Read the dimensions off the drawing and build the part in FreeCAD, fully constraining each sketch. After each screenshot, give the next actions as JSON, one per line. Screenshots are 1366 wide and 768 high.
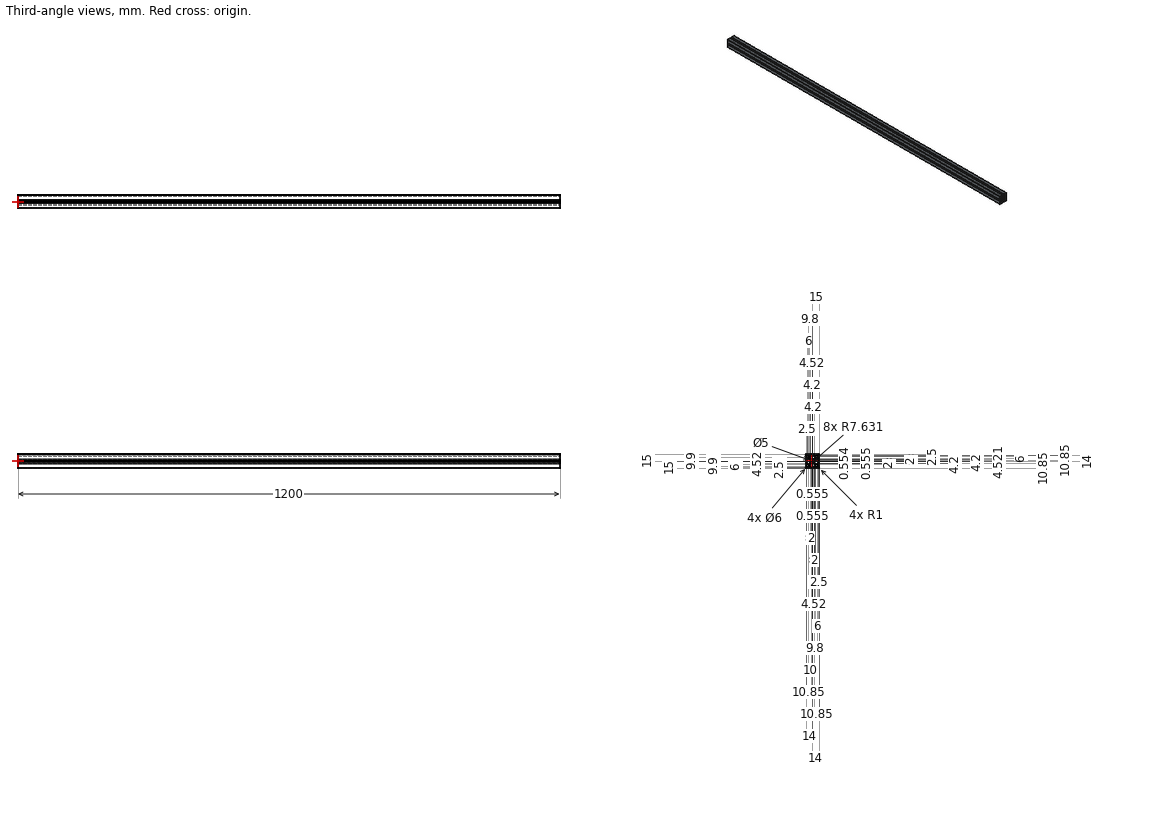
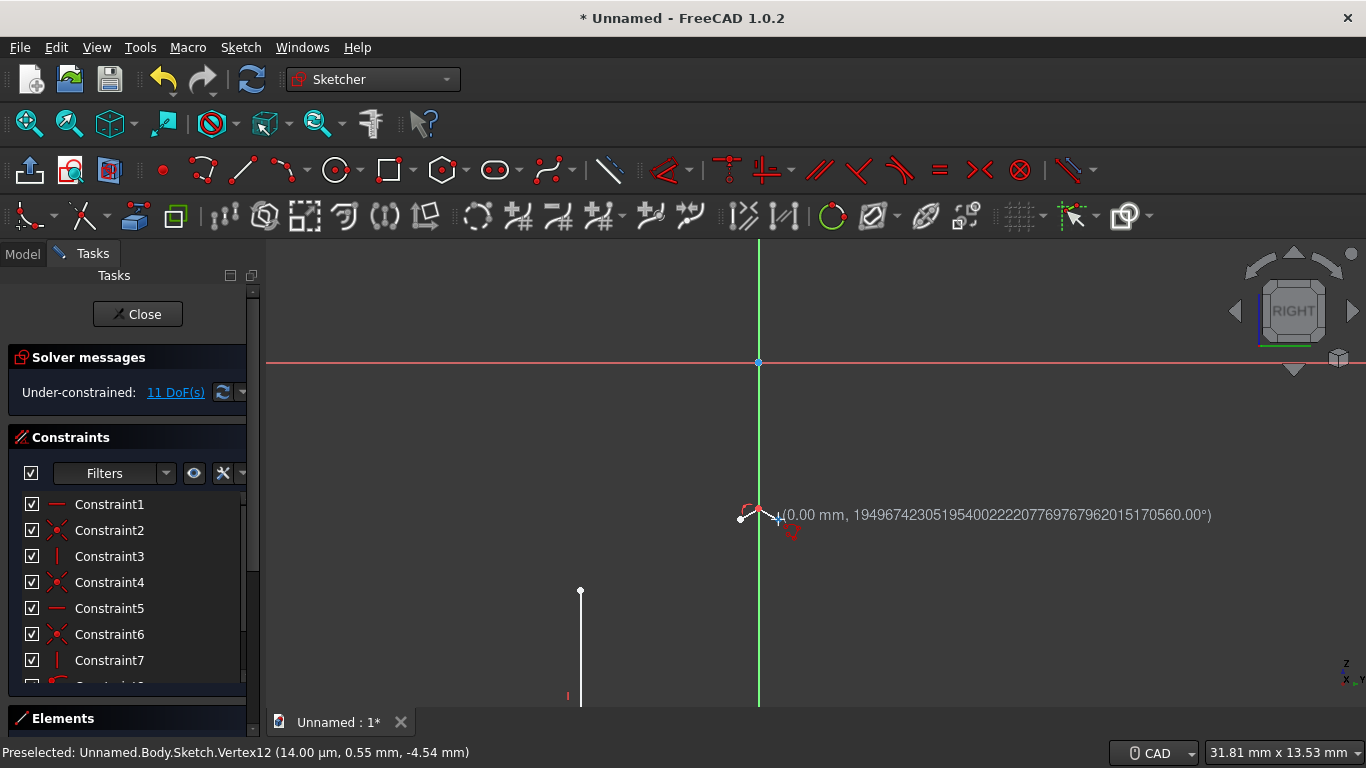
{"action": "left_click", "coordinate": [937, 588]}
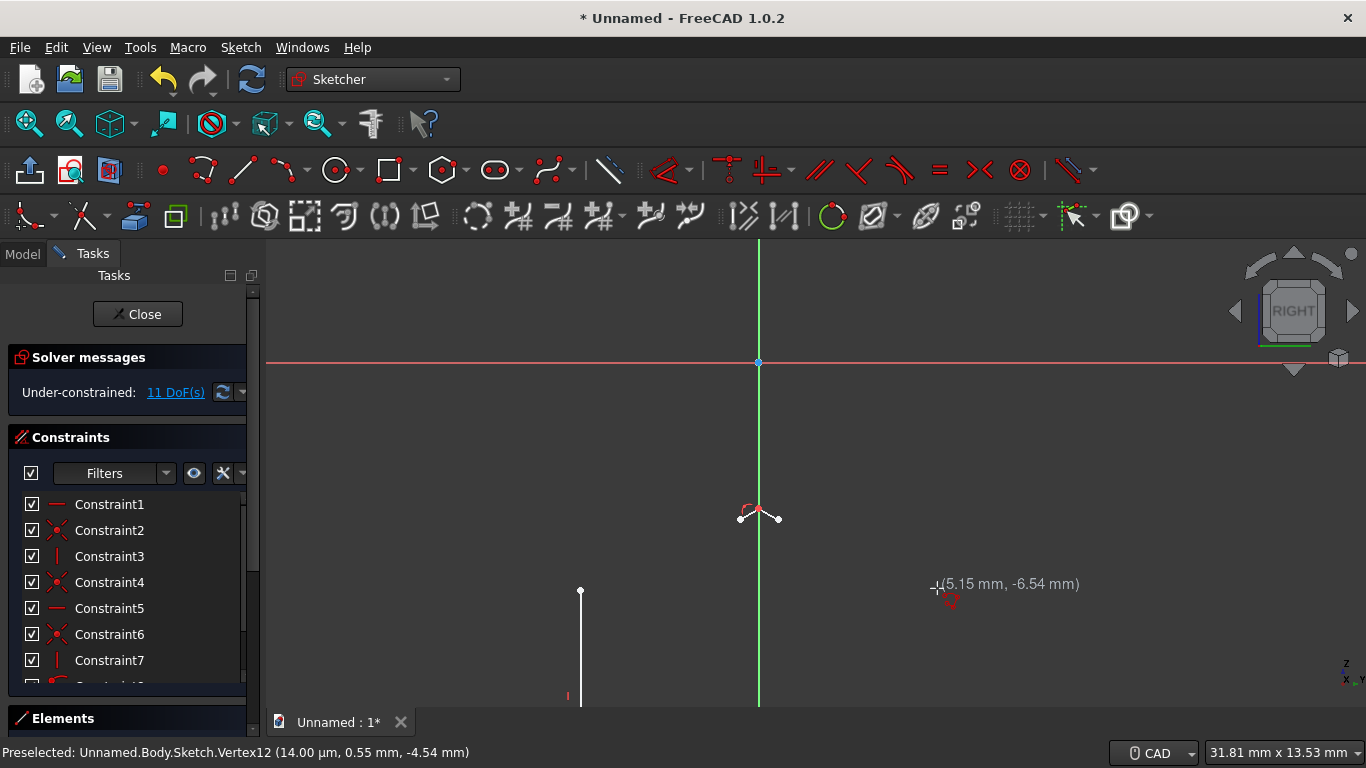
{"action": "scroll", "coordinate": [743, 520], "scroll_direction": "down", "scroll_amount": 6}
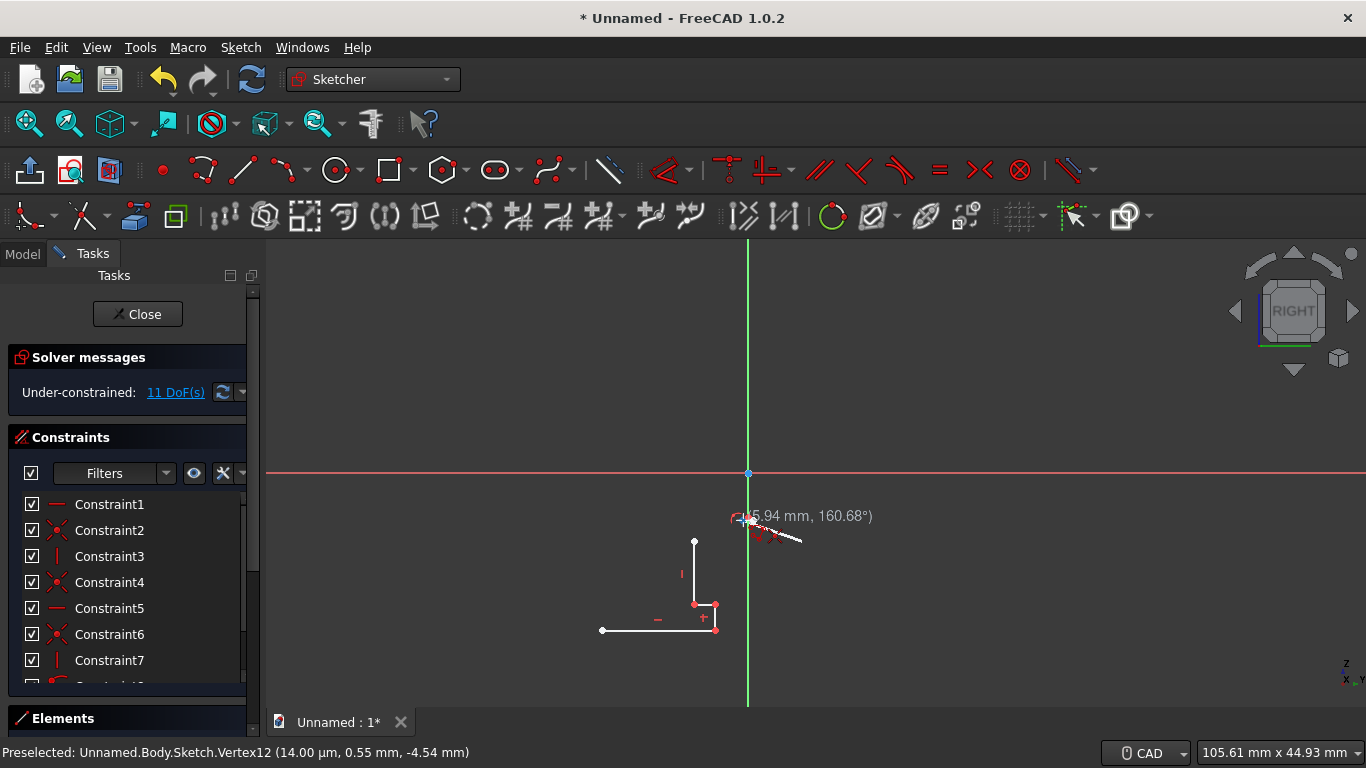
{"action": "left_click", "coordinate": [802, 603]}
{"action": "left_click", "coordinate": [781, 603]}
{"action": "left_click", "coordinate": [781, 629]}
{"action": "left_click", "coordinate": [894, 629]}
{"action": "right_click", "coordinate": [894, 629]}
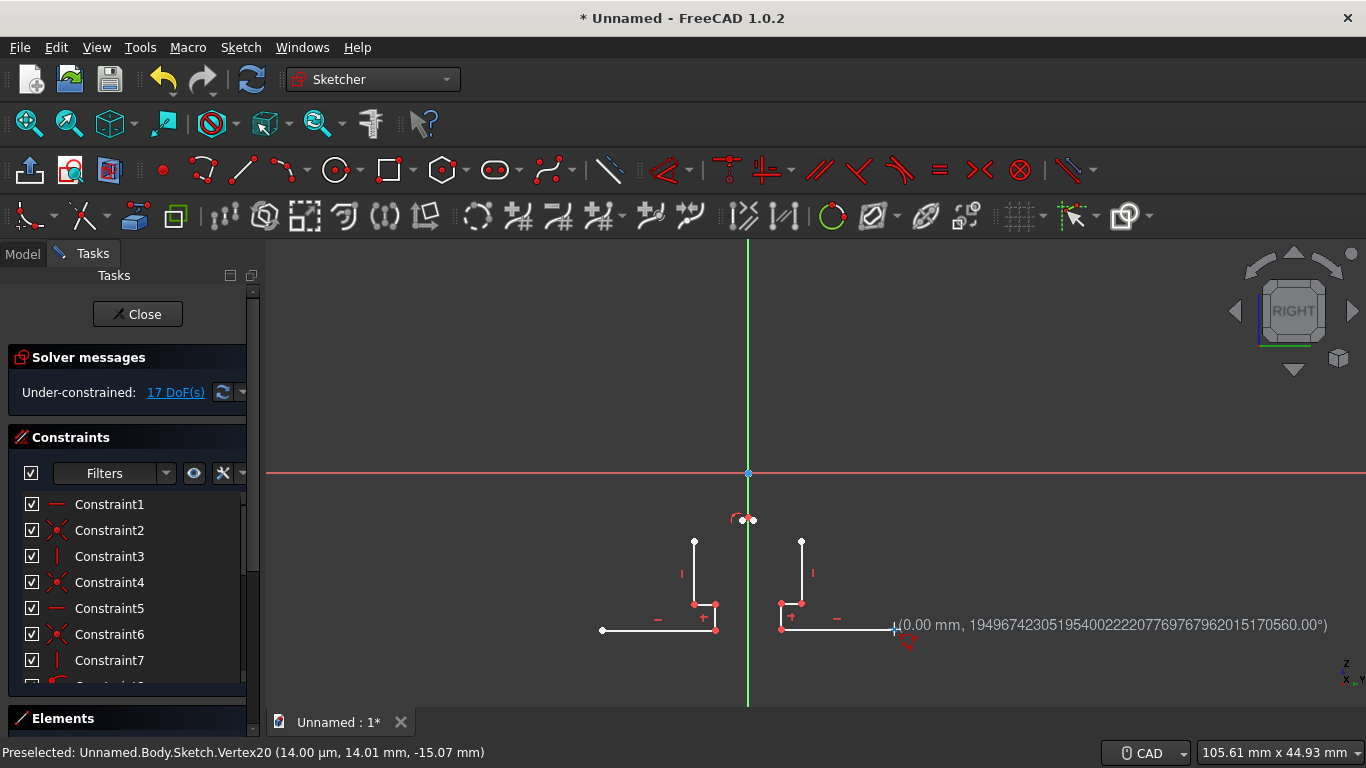
{"action": "left_click", "coordinate": [904, 619]}
{"action": "left_click", "coordinate": [904, 506]}
{"action": "left_click", "coordinate": [878, 506]}
{"action": "left_click", "coordinate": [878, 527]}
{"action": "left_click", "coordinate": [816, 527]}
{"action": "right_click", "coordinate": [816, 527]}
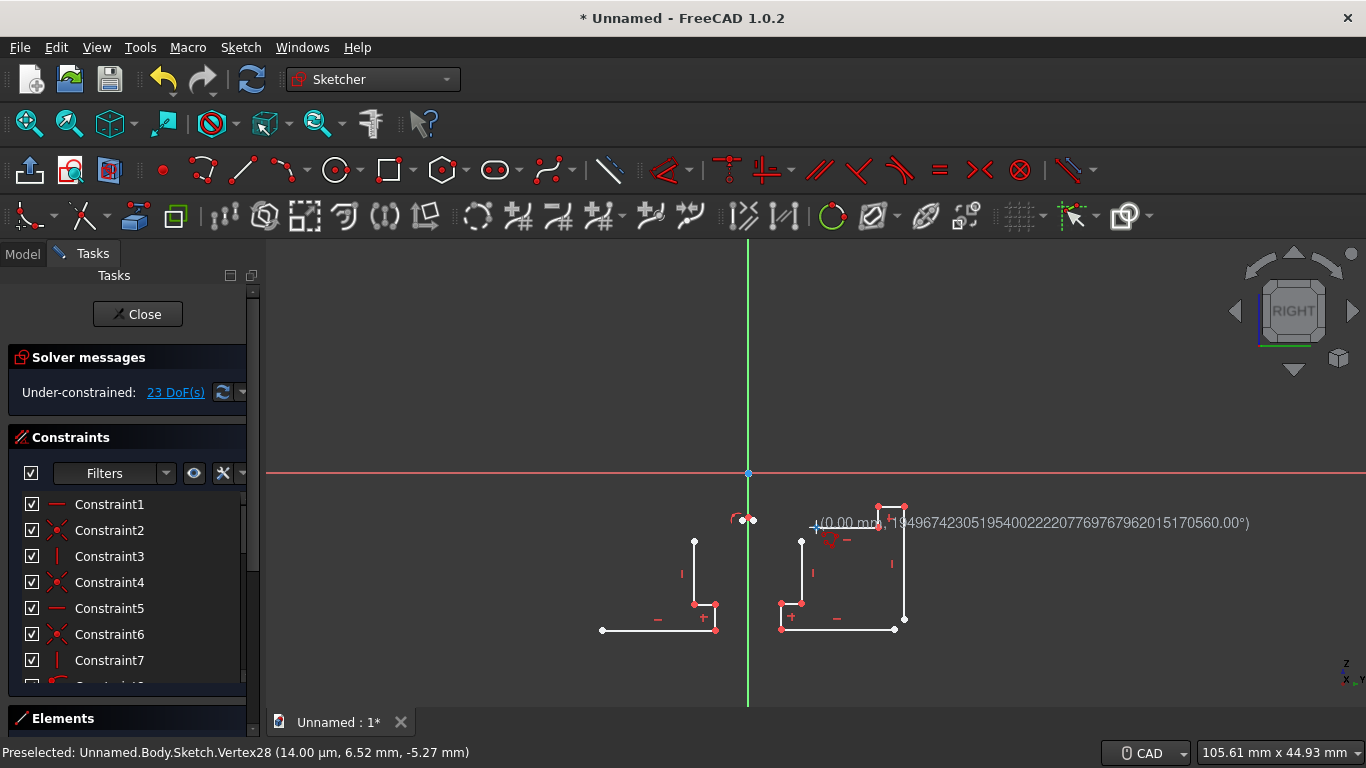
{"action": "scroll", "coordinate": [795, 479], "scroll_direction": "up", "scroll_amount": 6}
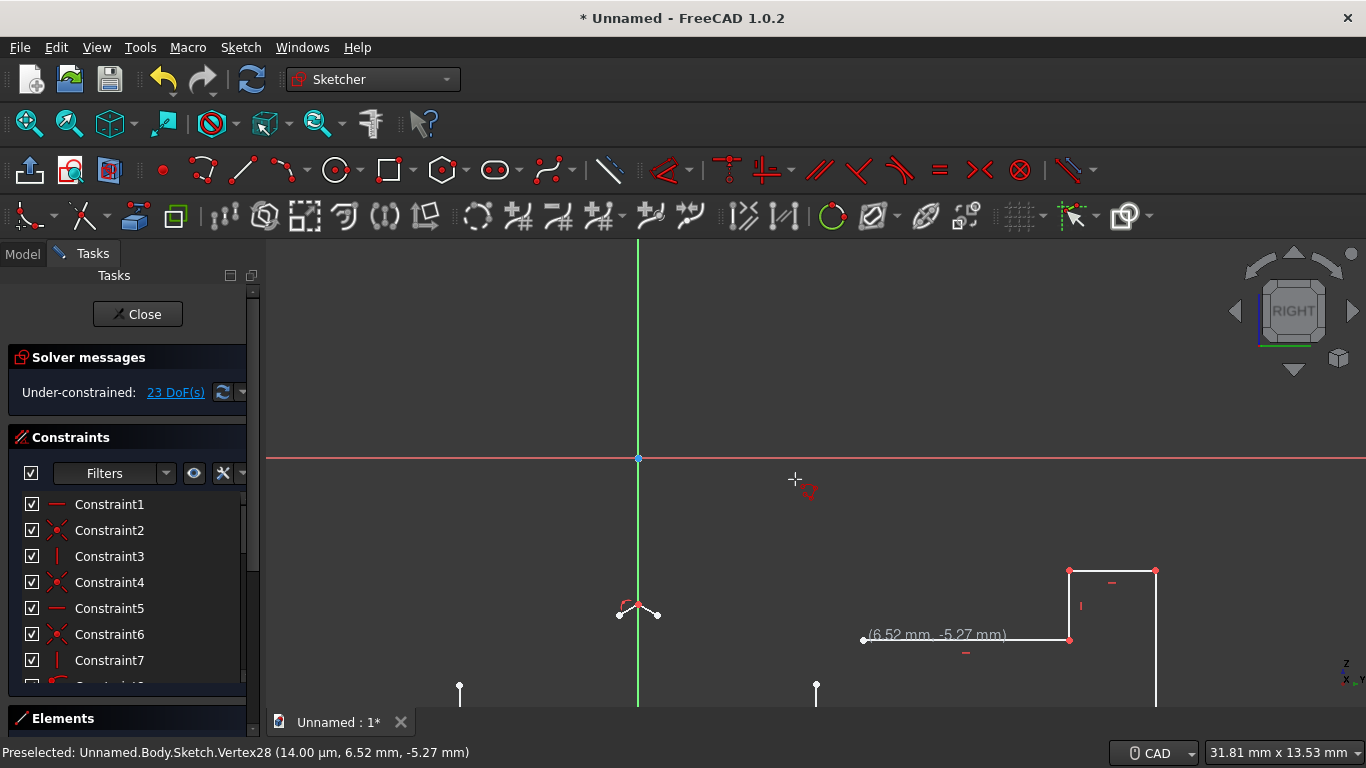
{"action": "left_click", "coordinate": [794, 477]}
{"action": "left_click", "coordinate": [783, 458]}
{"action": "left_click", "coordinate": [794, 439]}
{"action": "right_click", "coordinate": [794, 439]}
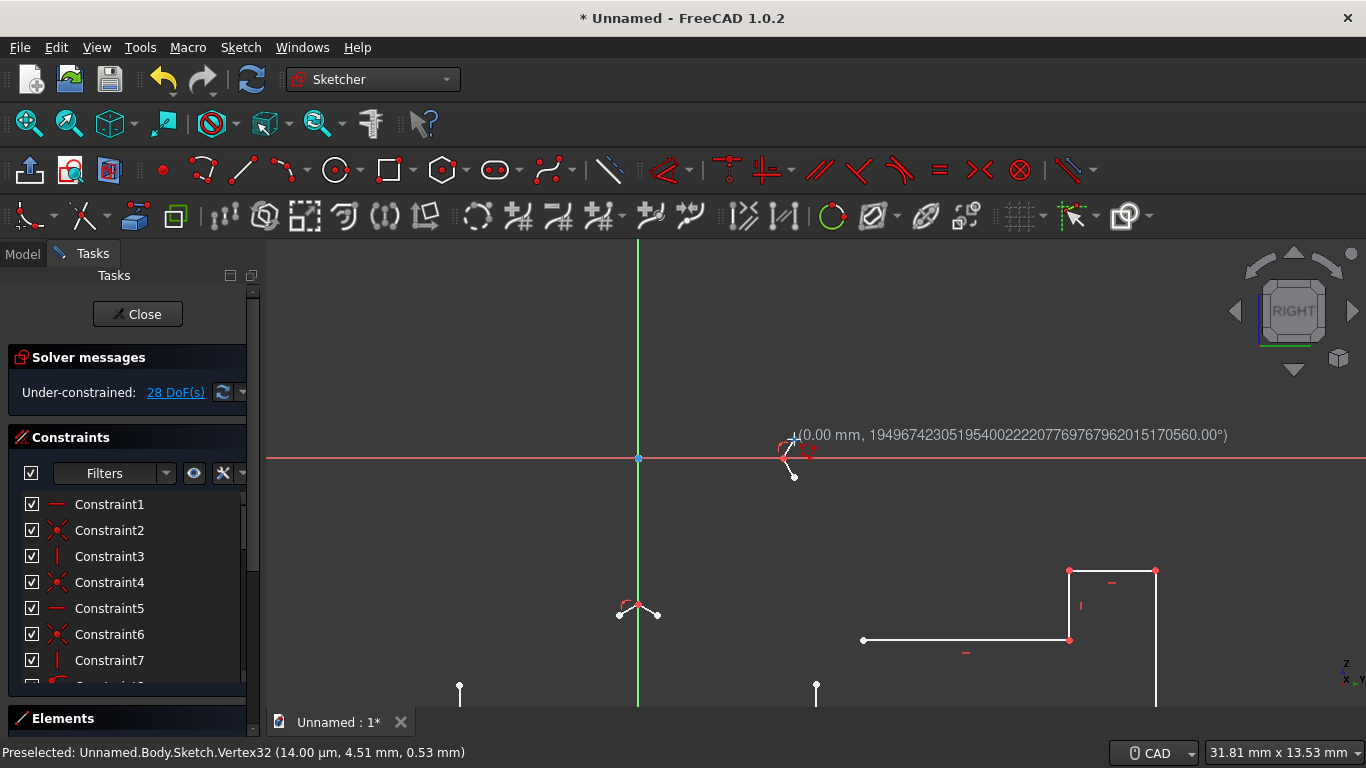
{"action": "left_click", "coordinate": [863, 280]}
{"action": "left_click", "coordinate": [1070, 280]}
{"action": "left_click", "coordinate": [1070, 349]}
{"action": "left_click", "coordinate": [1157, 349]}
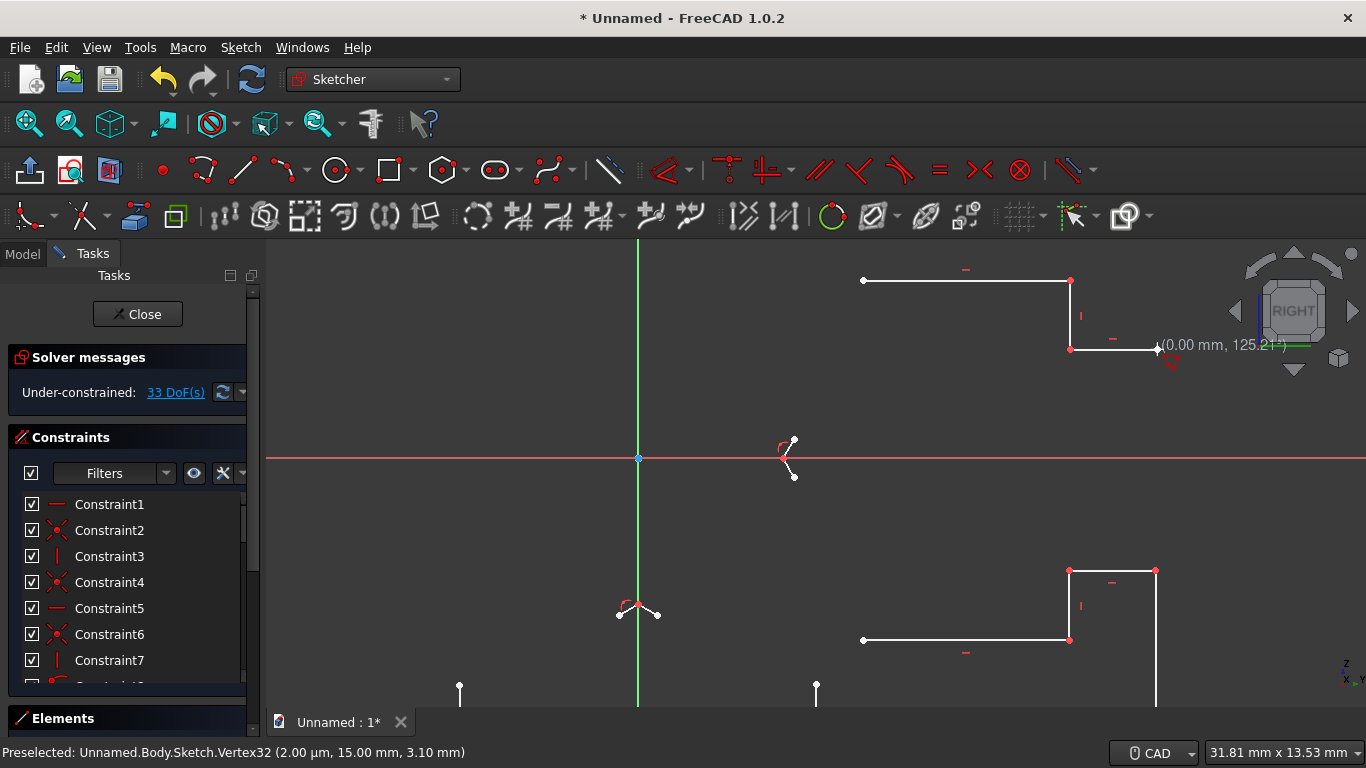
{"action": "scroll", "coordinate": [795, 479], "scroll_direction": "down", "scroll_amount": 6}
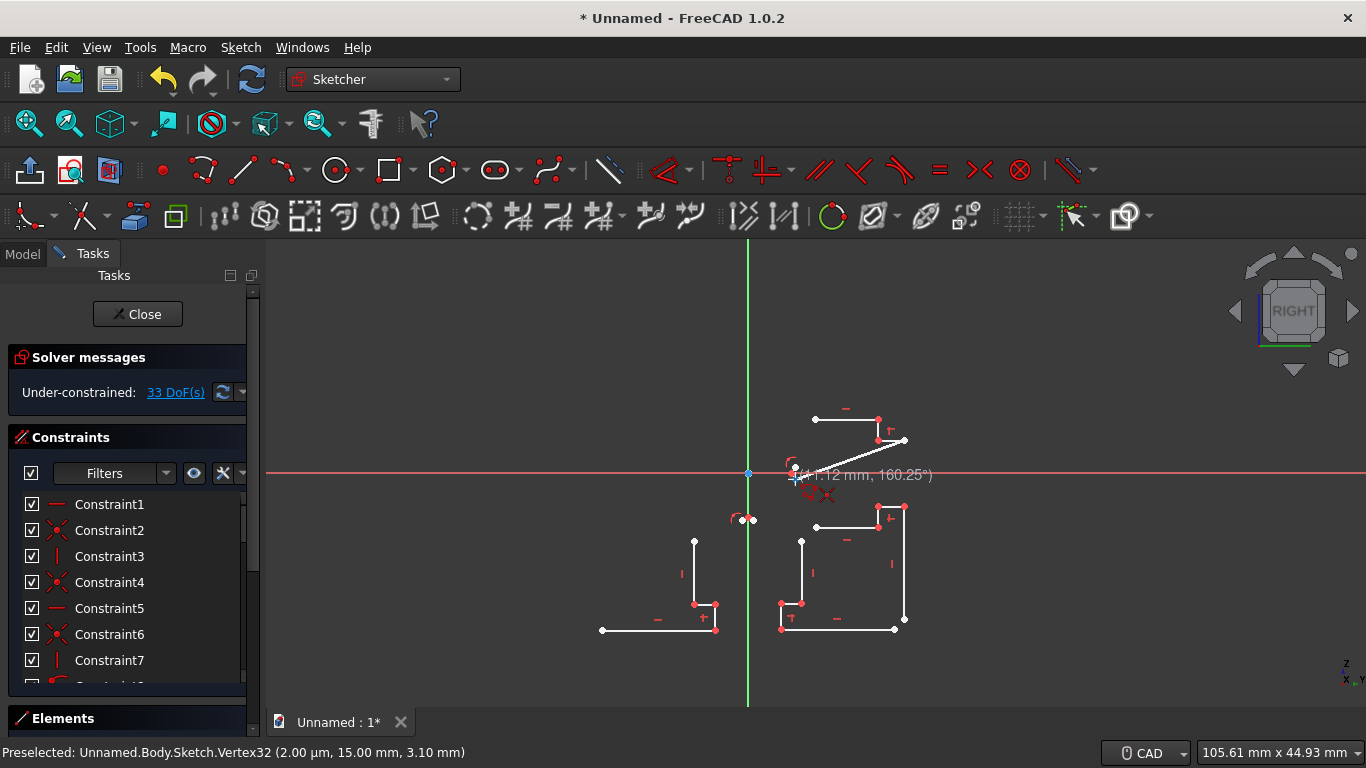
{"action": "left_click", "coordinate": [904, 327]}
{"action": "right_click", "coordinate": [904, 327]}